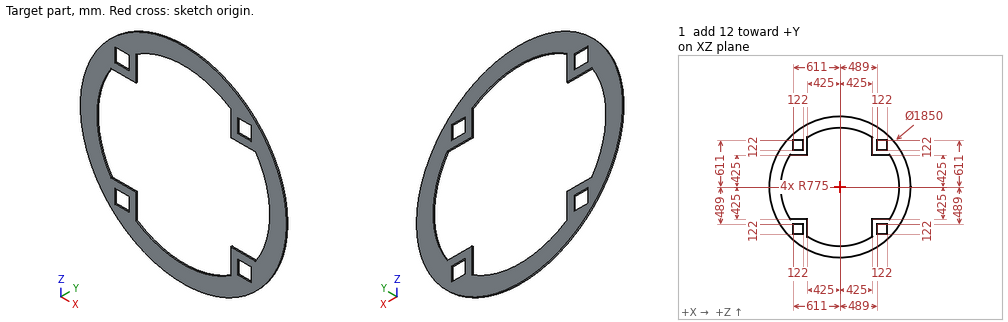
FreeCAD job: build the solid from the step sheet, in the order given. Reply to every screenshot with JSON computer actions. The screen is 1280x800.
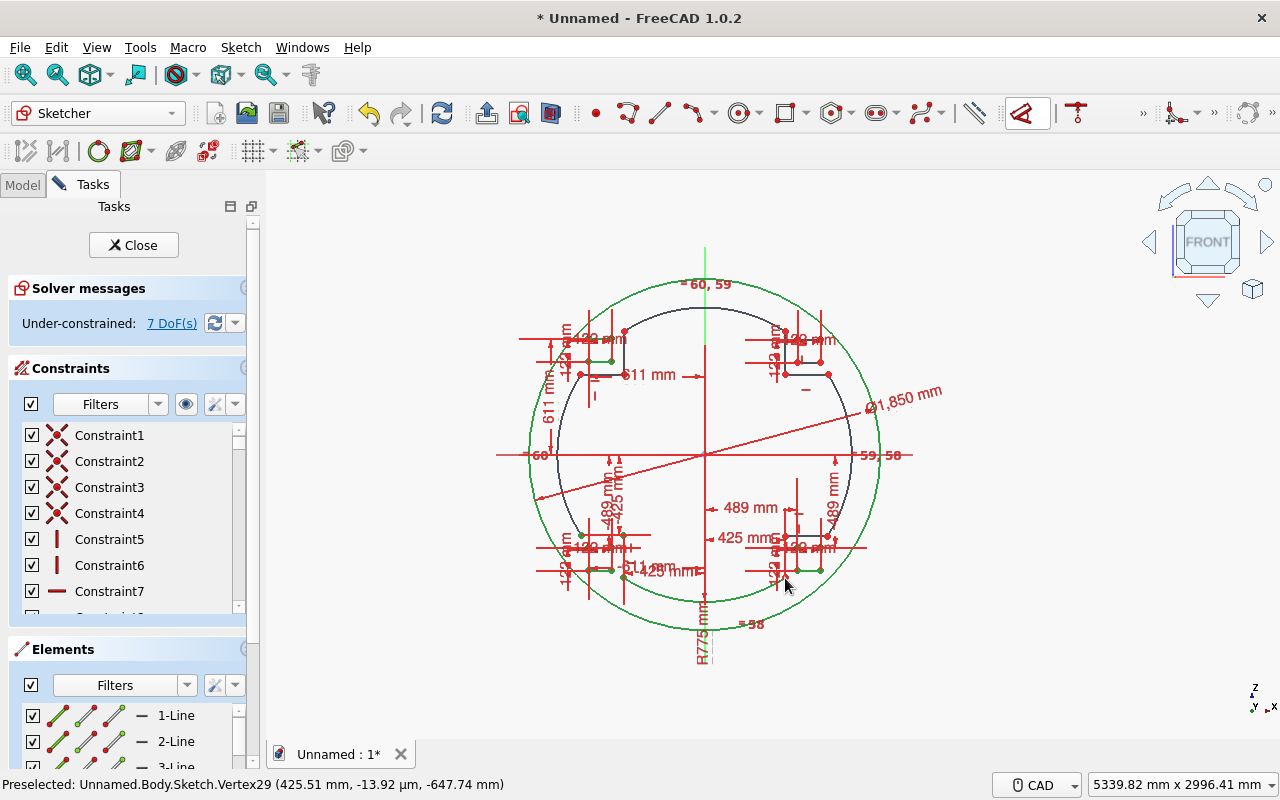
{"action": "left_click", "coordinate": [785, 536]}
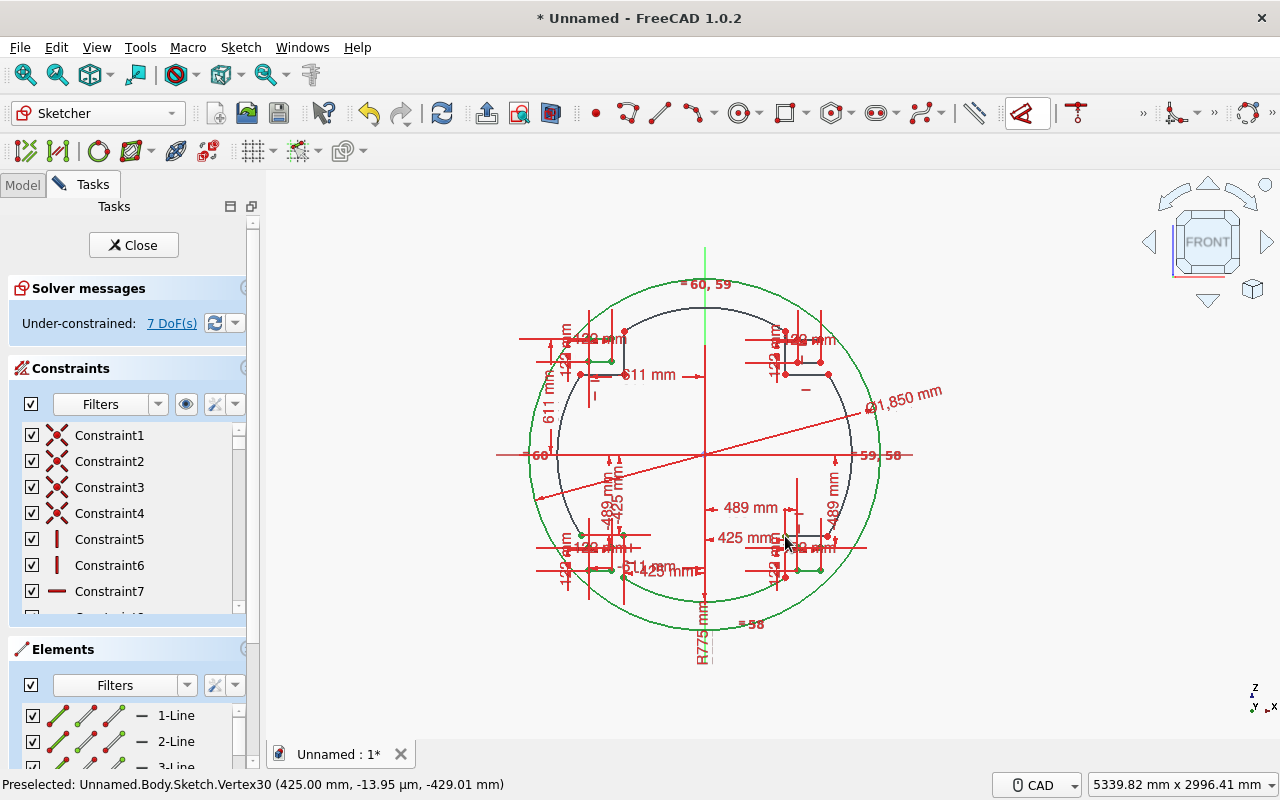
{"action": "left_click", "coordinate": [1044, 114]}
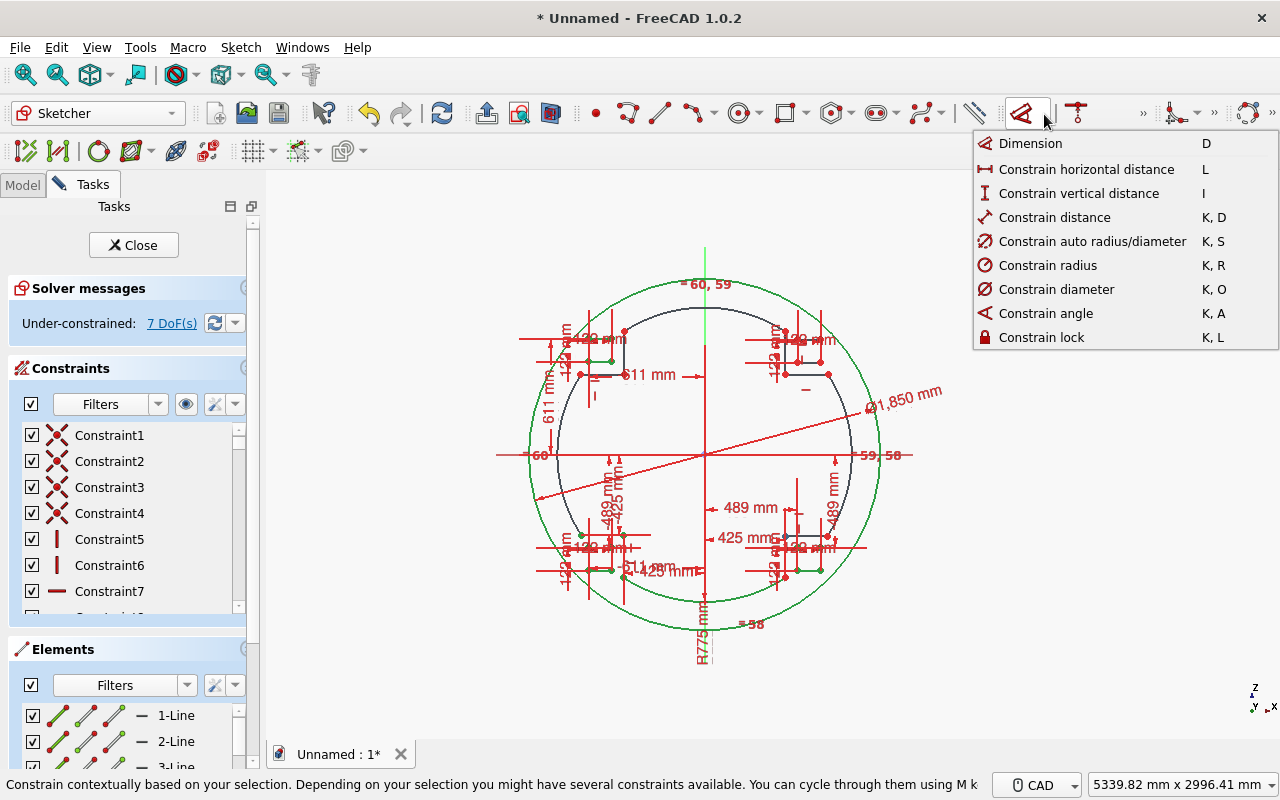
{"action": "left_click", "coordinate": [1126, 193]}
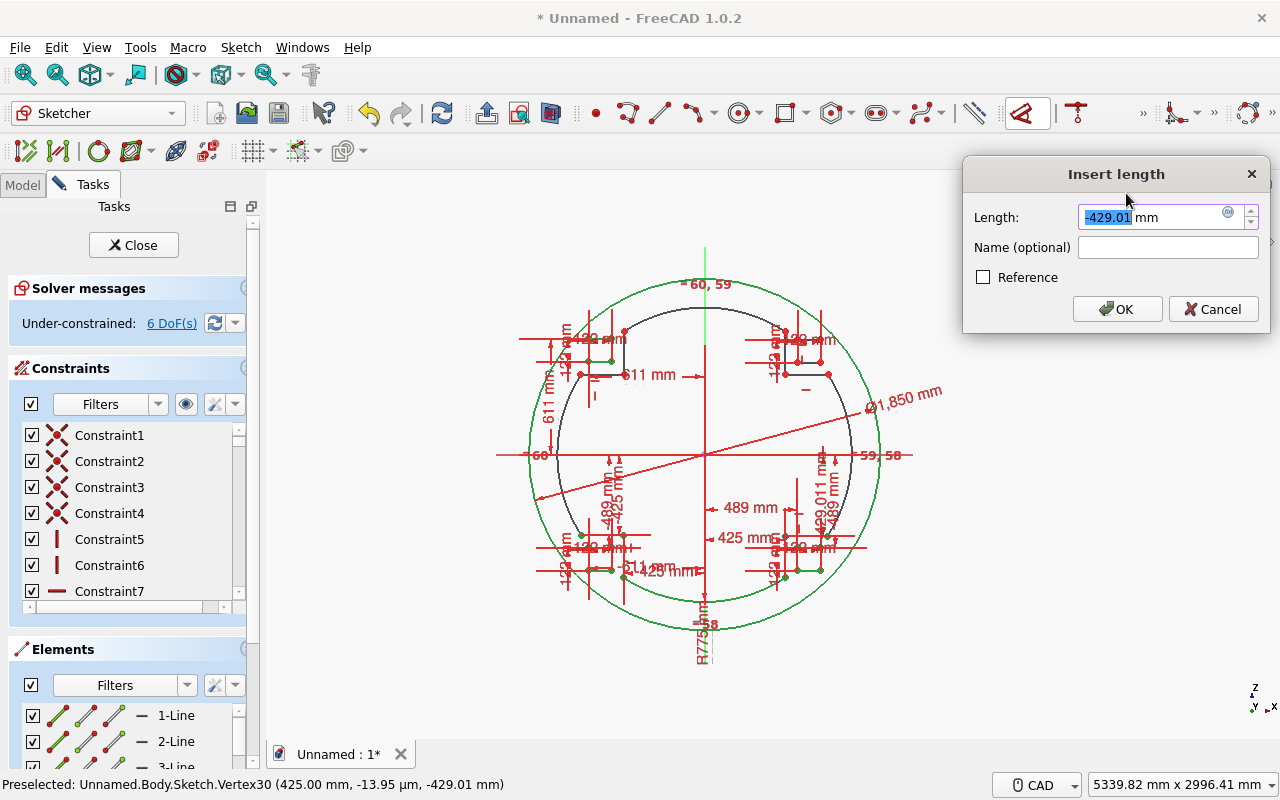
{"action": "type", "text": "-425"}
{"action": "key", "text": "Return"}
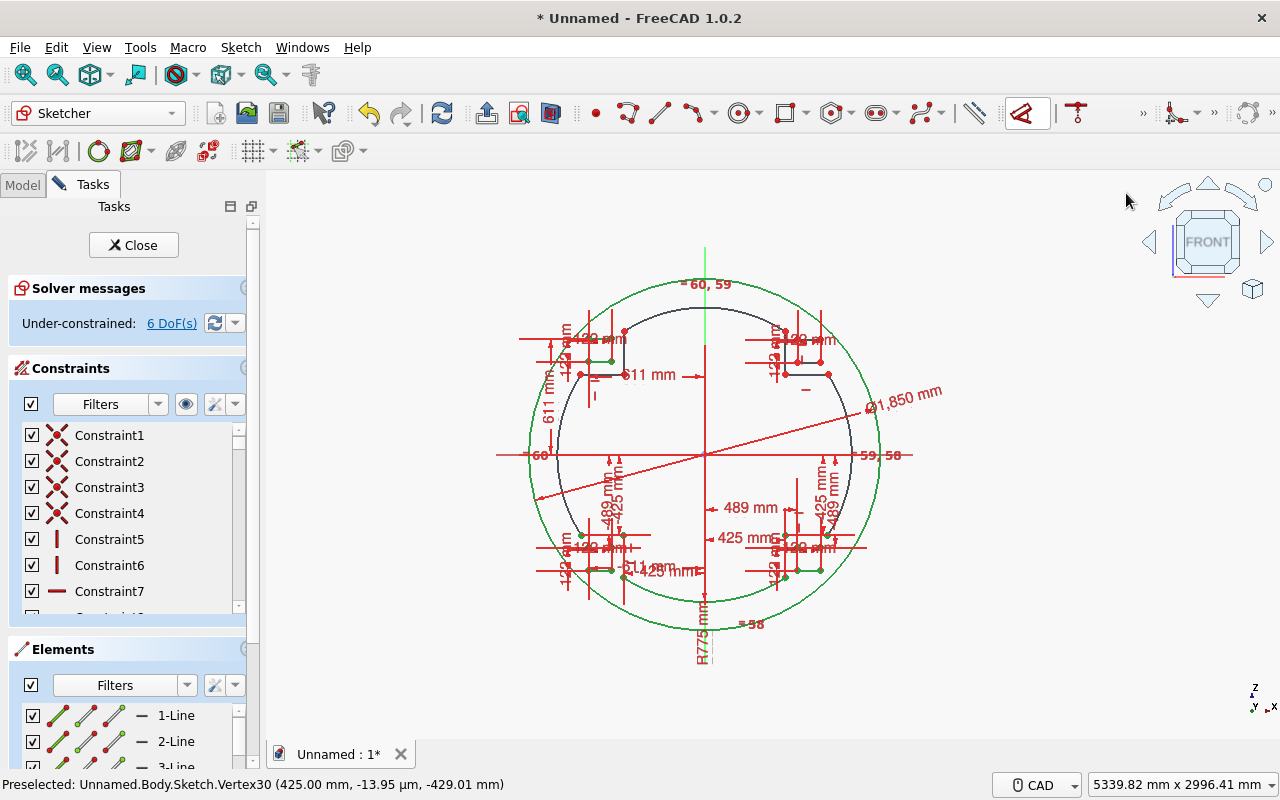
{"action": "left_click", "coordinate": [828, 375]}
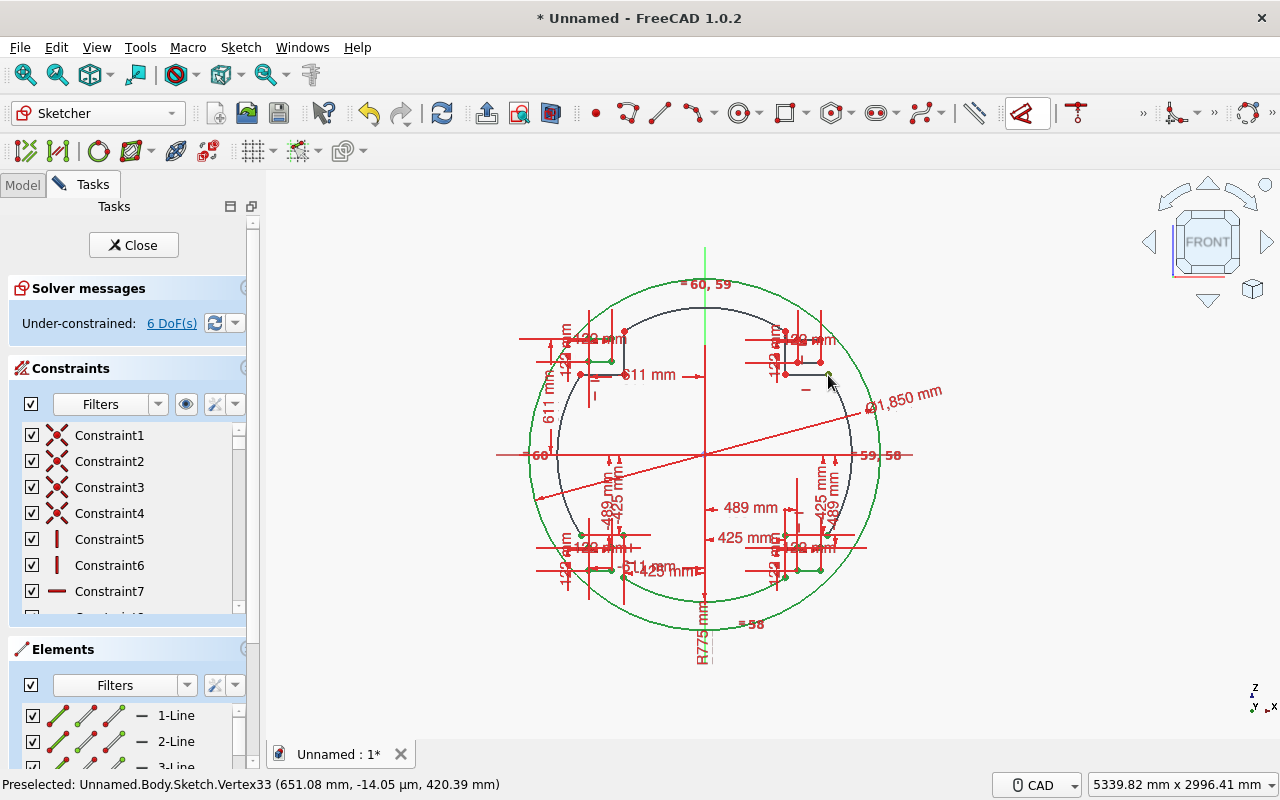
{"action": "key", "text": "i"}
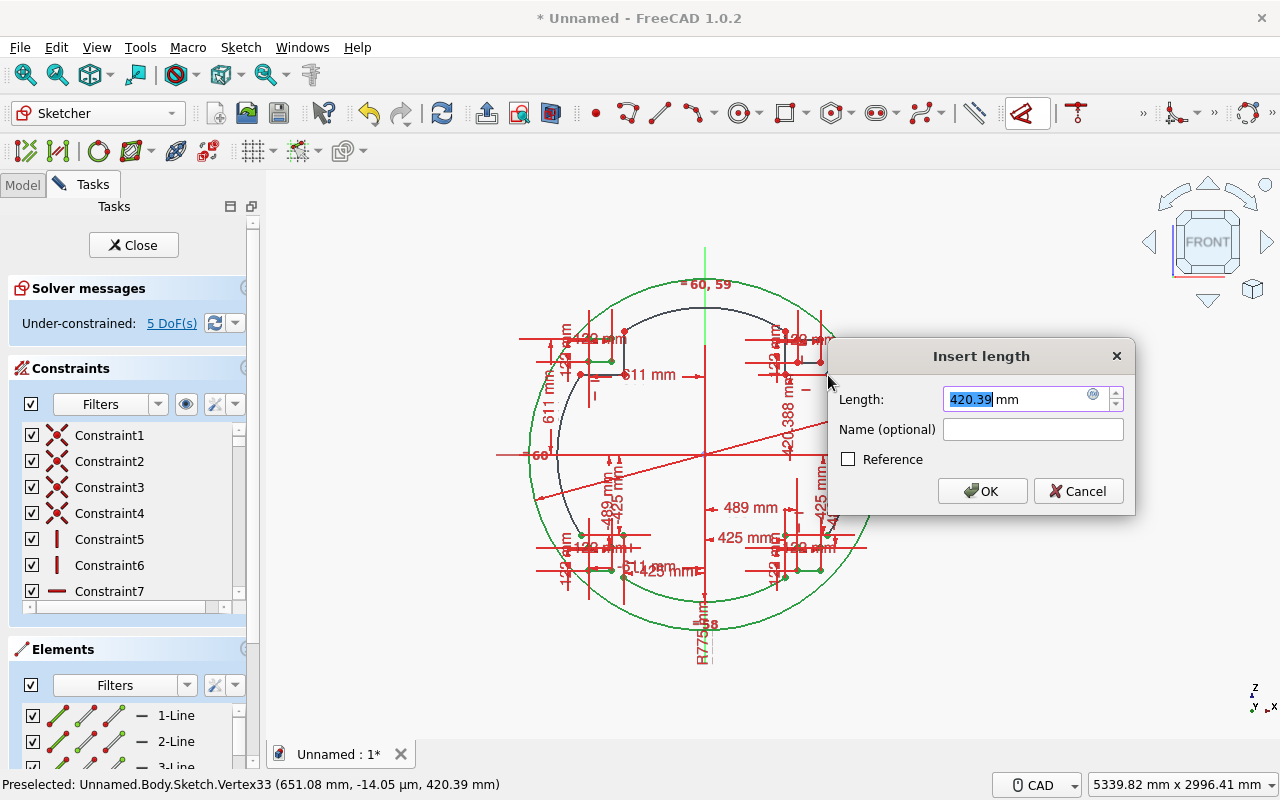
{"action": "type", "text": "425"}
{"action": "key", "text": "Return"}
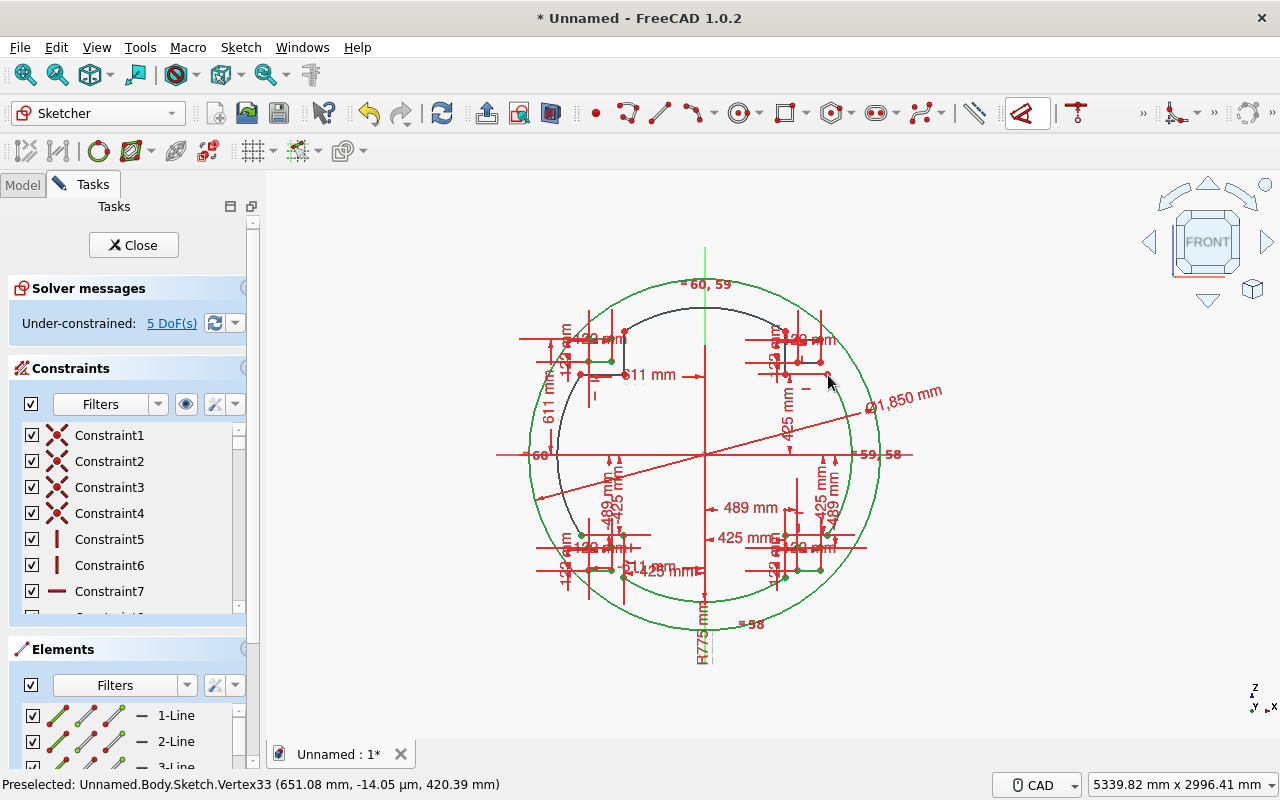
{"action": "left_click", "coordinate": [785, 374]}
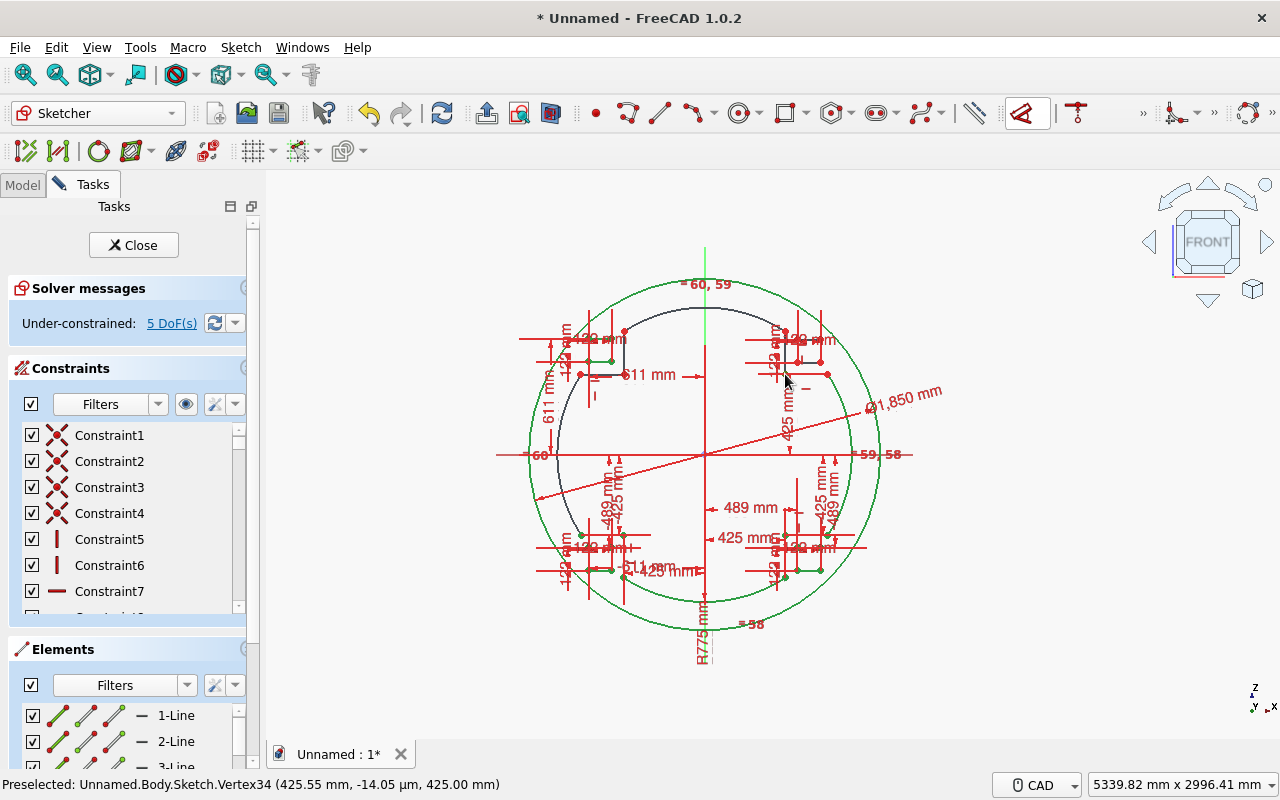
{"action": "key", "text": "l"}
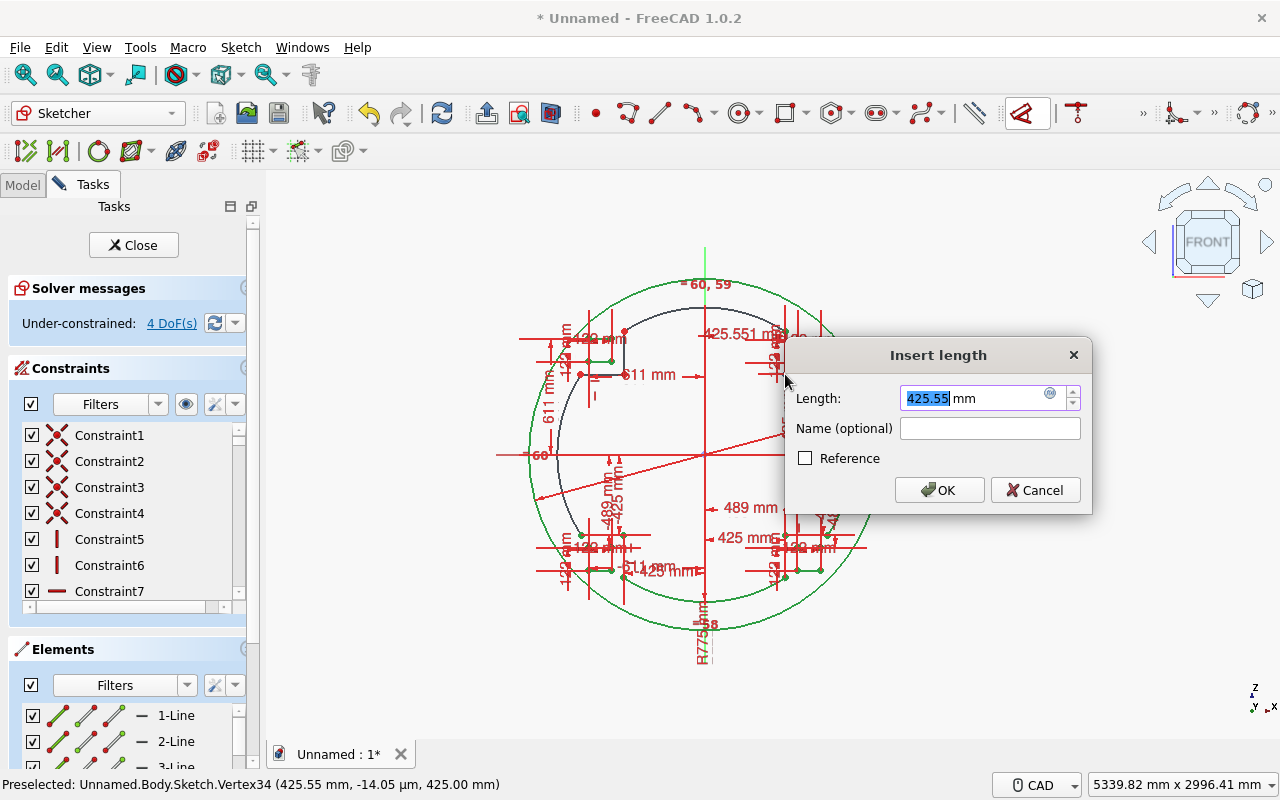
{"action": "type", "text": "425"}
{"action": "key", "text": "Return"}